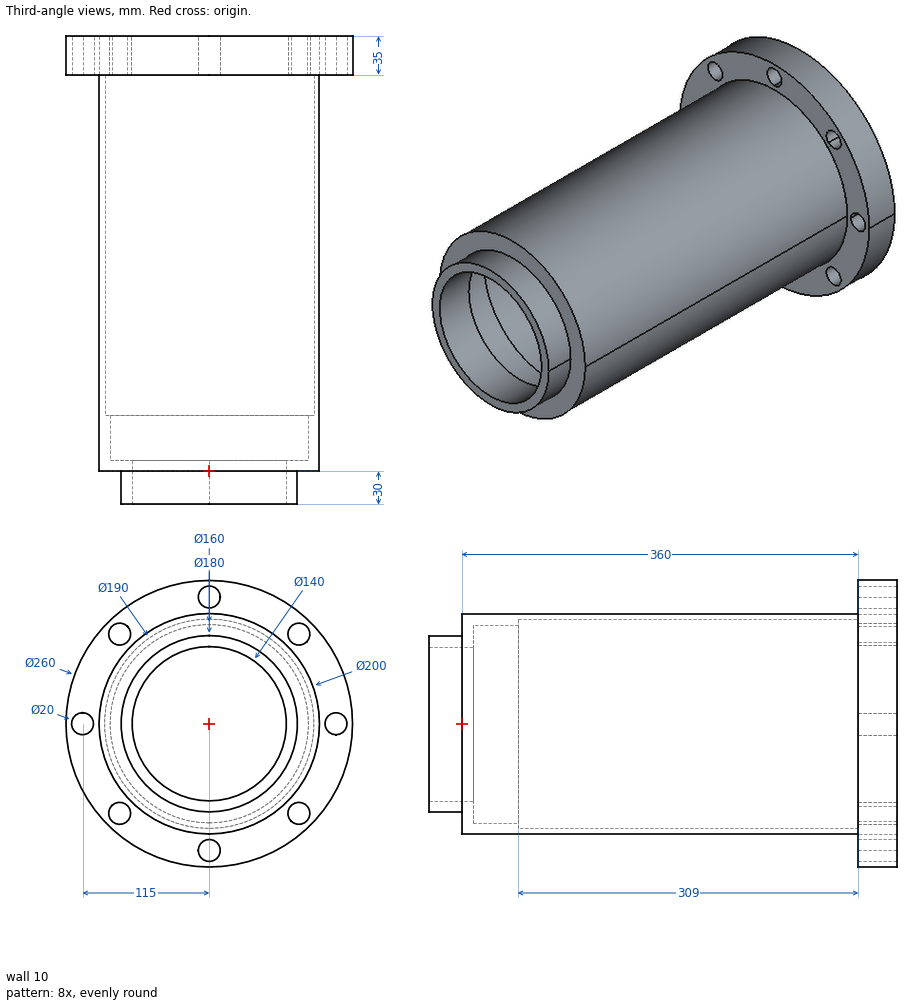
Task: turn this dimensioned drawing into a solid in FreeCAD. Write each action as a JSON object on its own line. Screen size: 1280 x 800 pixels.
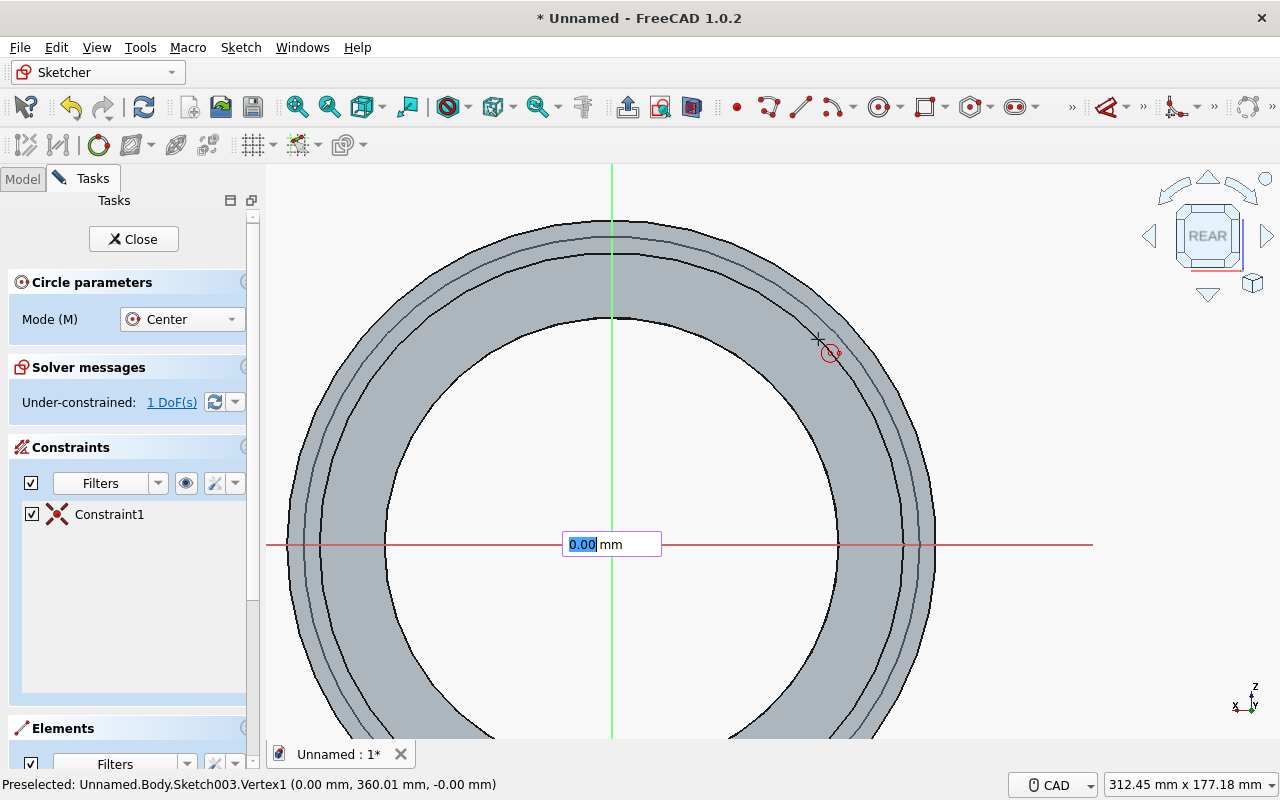
{"action": "left_click", "coordinate": [818, 338]}
{"action": "key", "text": "Escape"}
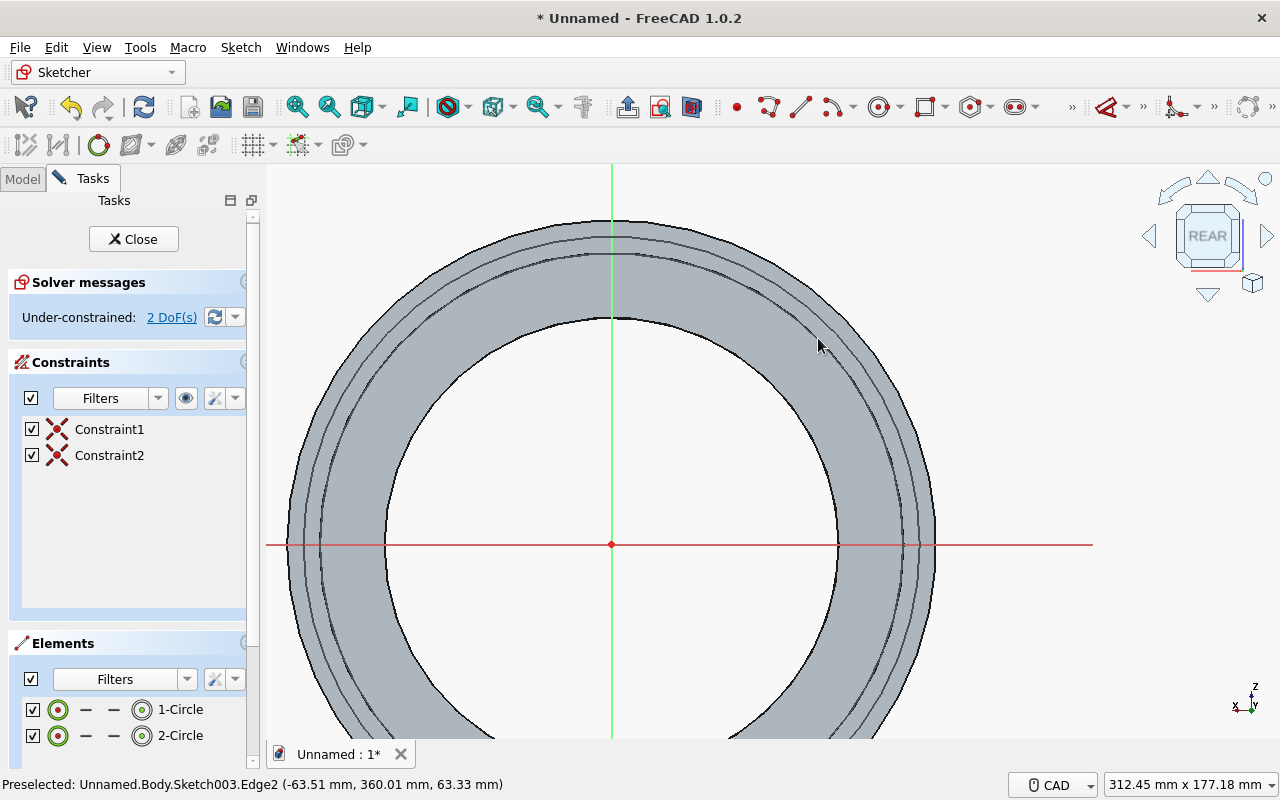
{"action": "left_click", "coordinate": [1106, 108]}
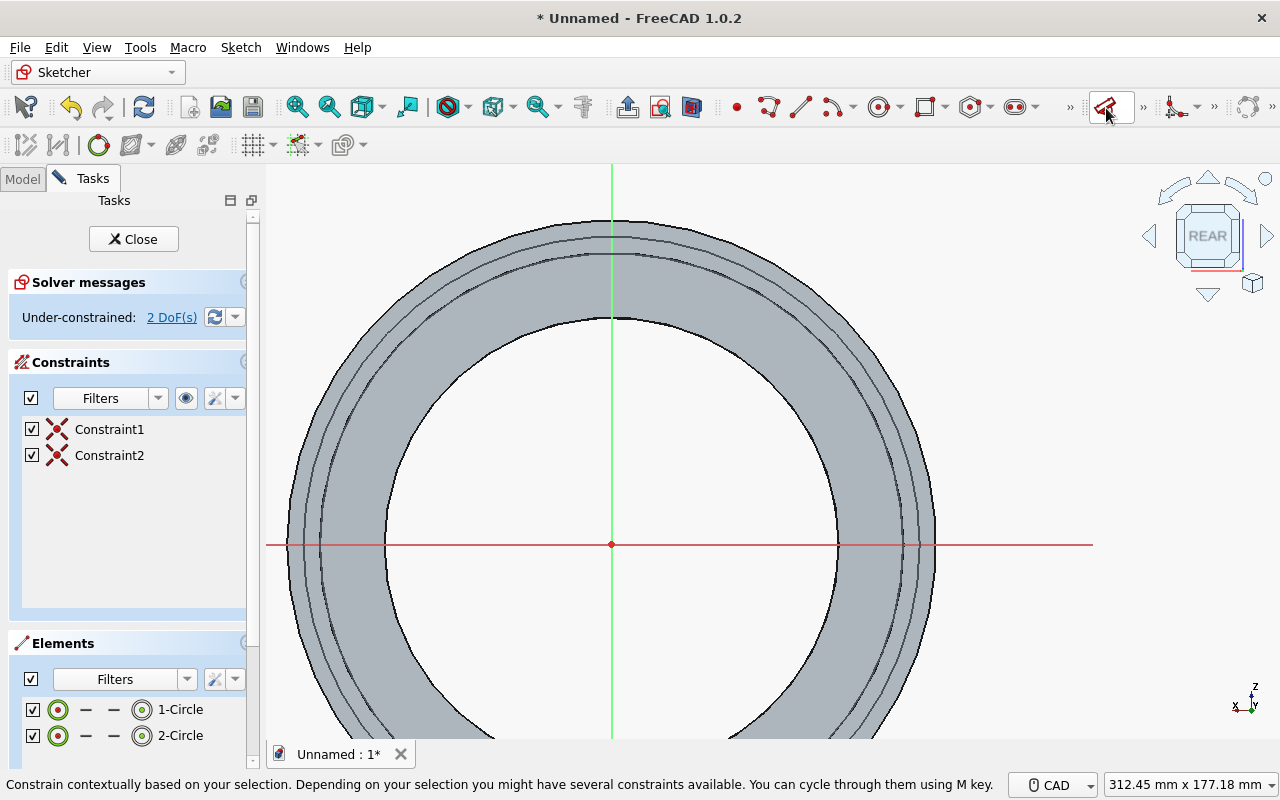
{"action": "left_click", "coordinate": [829, 326]}
{"action": "left_click", "coordinate": [852, 303]}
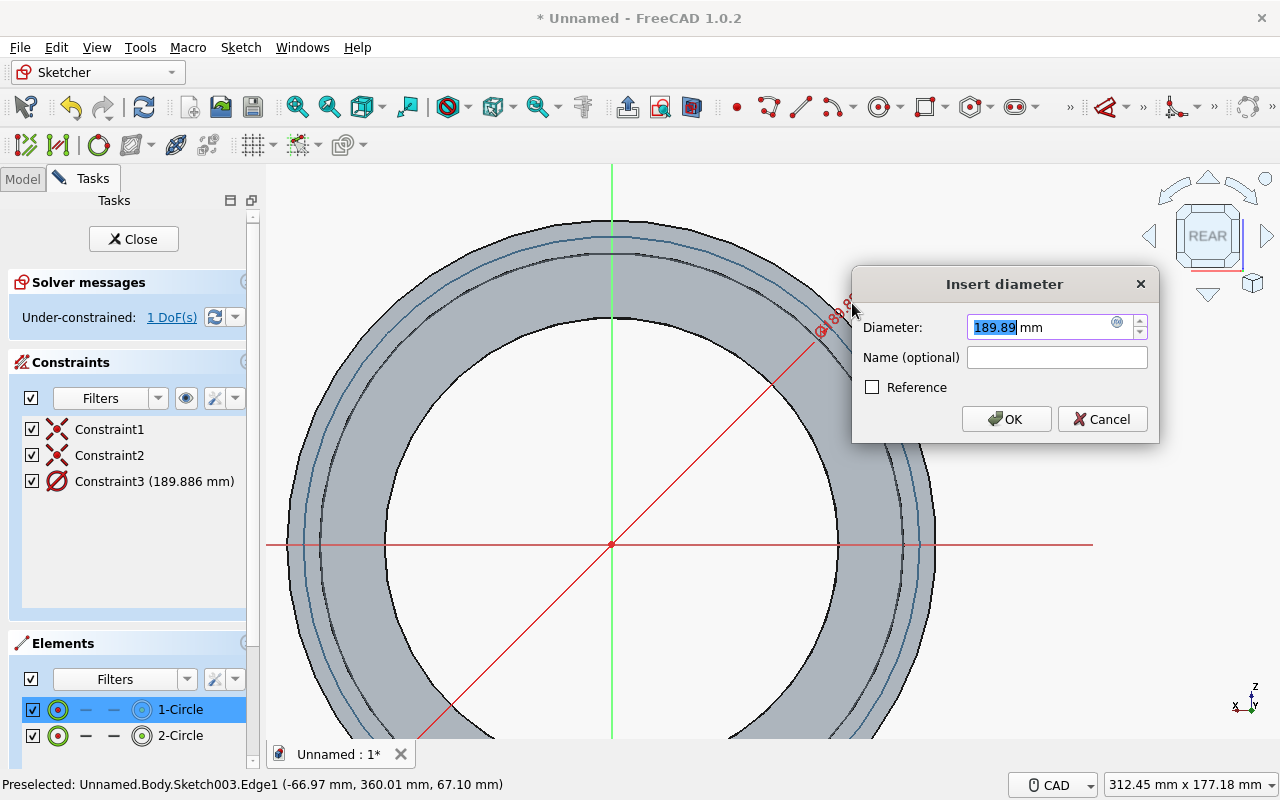
{"action": "type", "text": "190"}
{"action": "key", "text": "Return"}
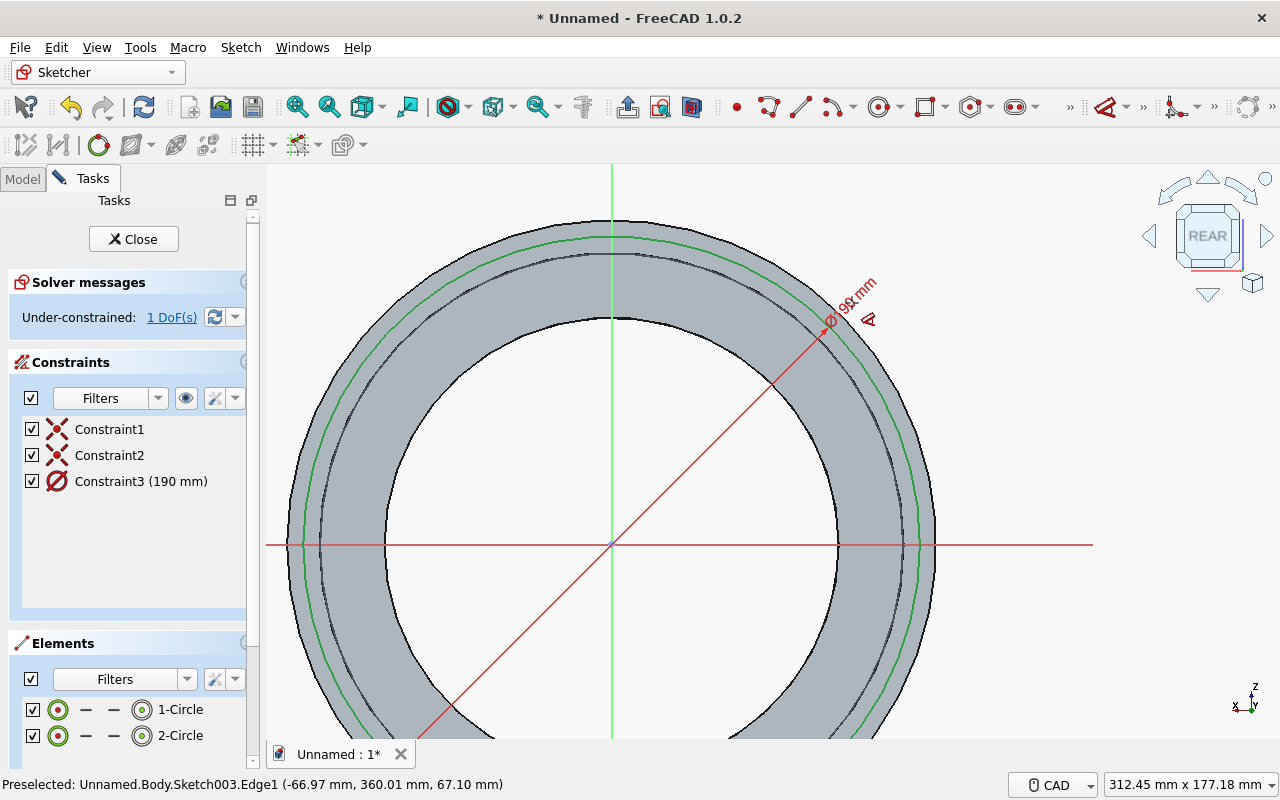
{"action": "left_click", "coordinate": [817, 338]}
{"action": "left_click", "coordinate": [922, 453]}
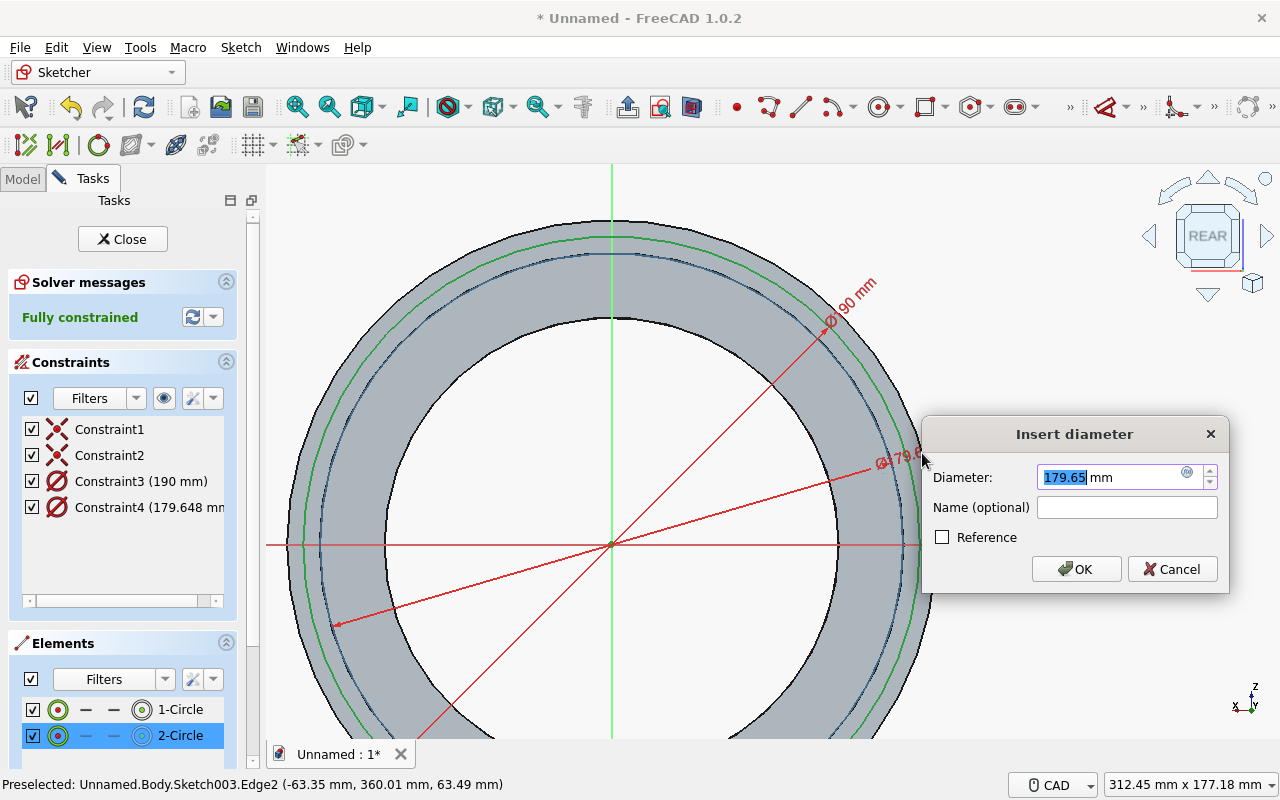
{"action": "type", "text": "180"}
{"action": "key", "text": "Return"}
{"action": "key", "text": "Escape"}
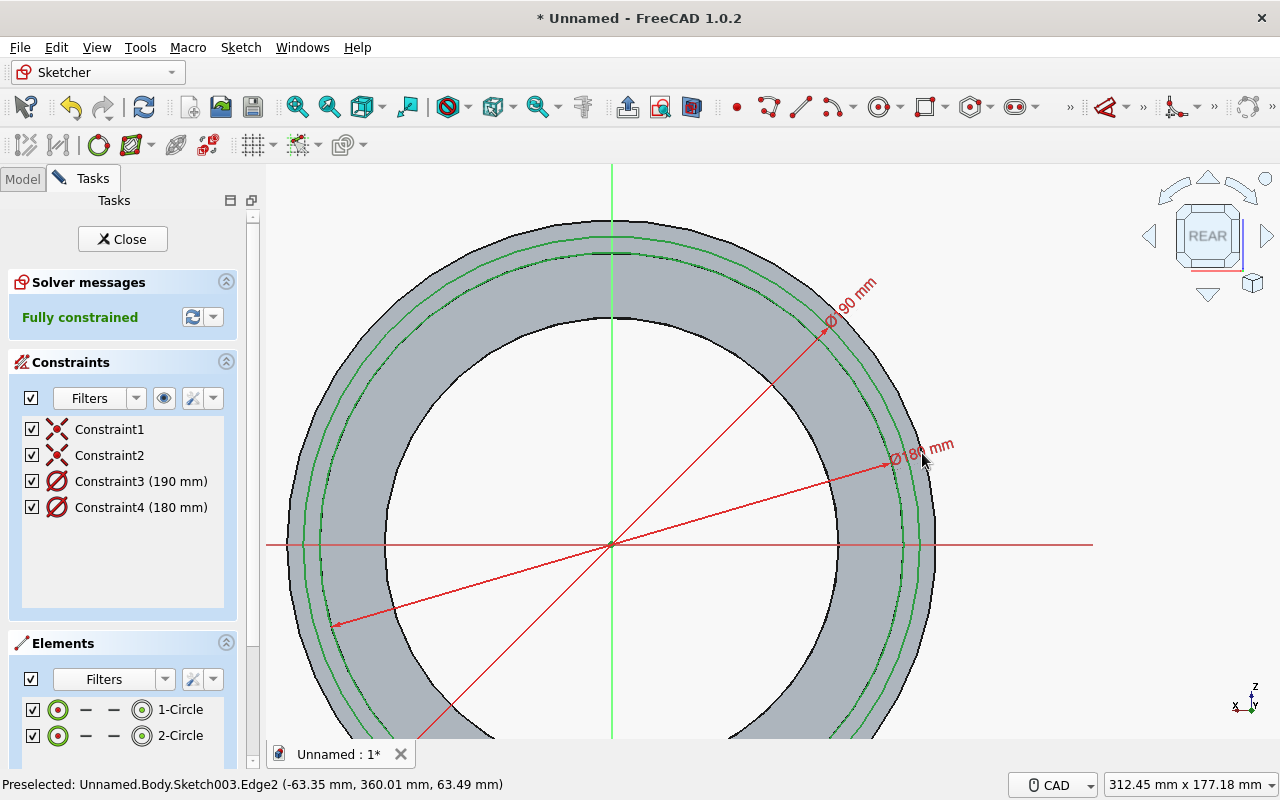
{"action": "left_click", "coordinate": [123, 239]}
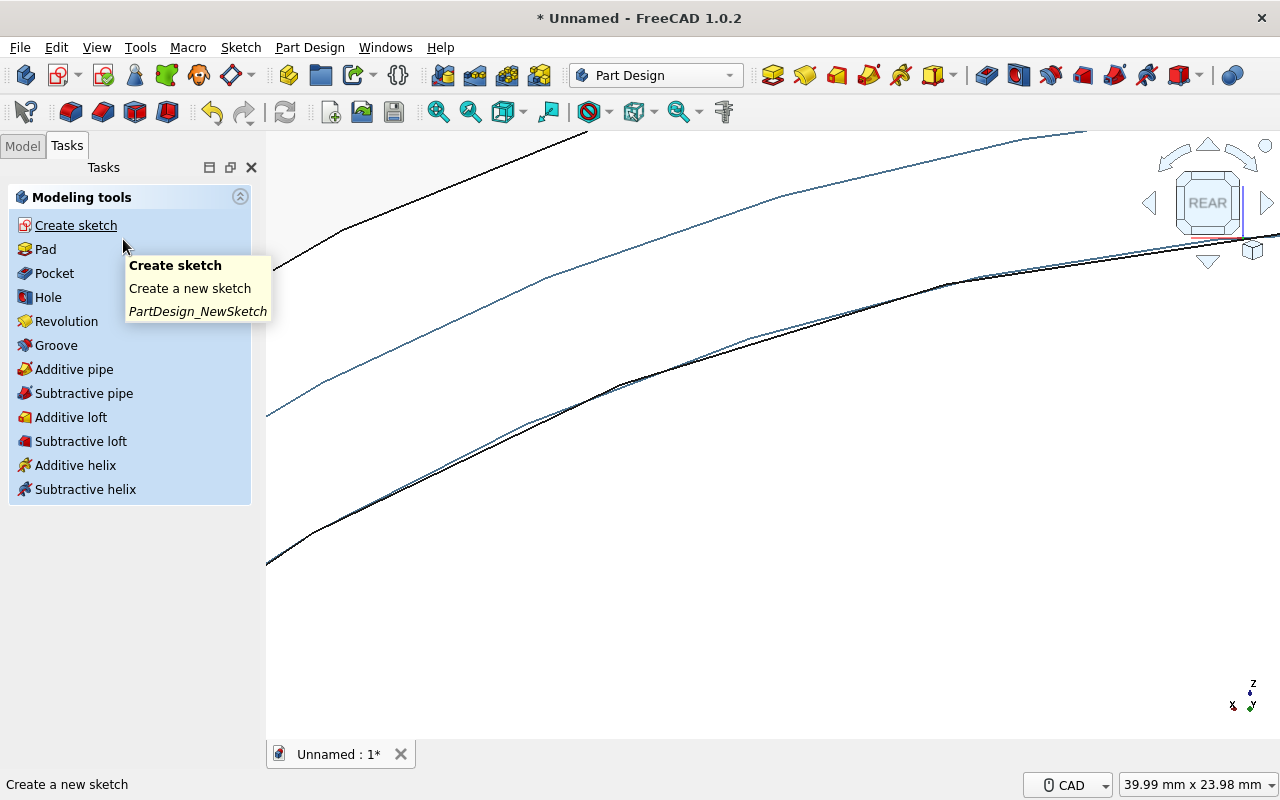
{"action": "left_click", "coordinate": [988, 76]}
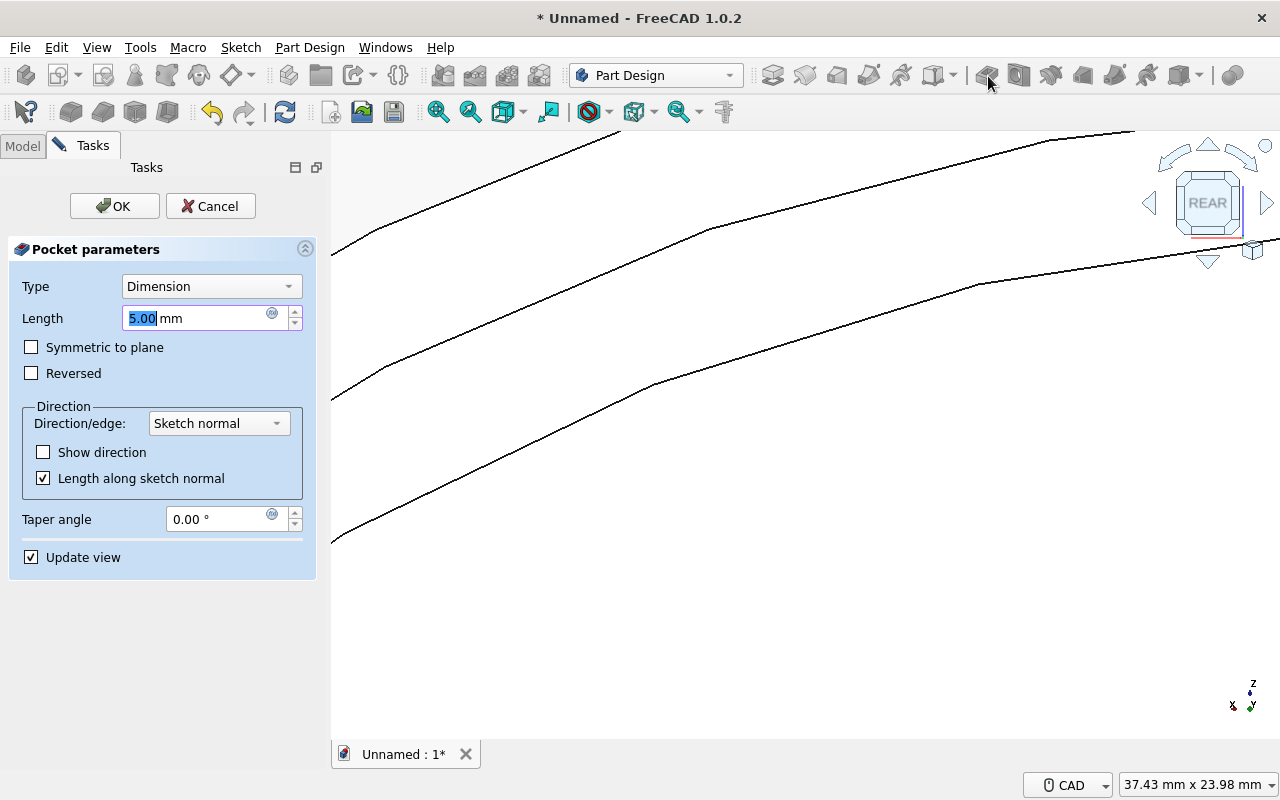
{"action": "left_click", "coordinate": [212, 286]}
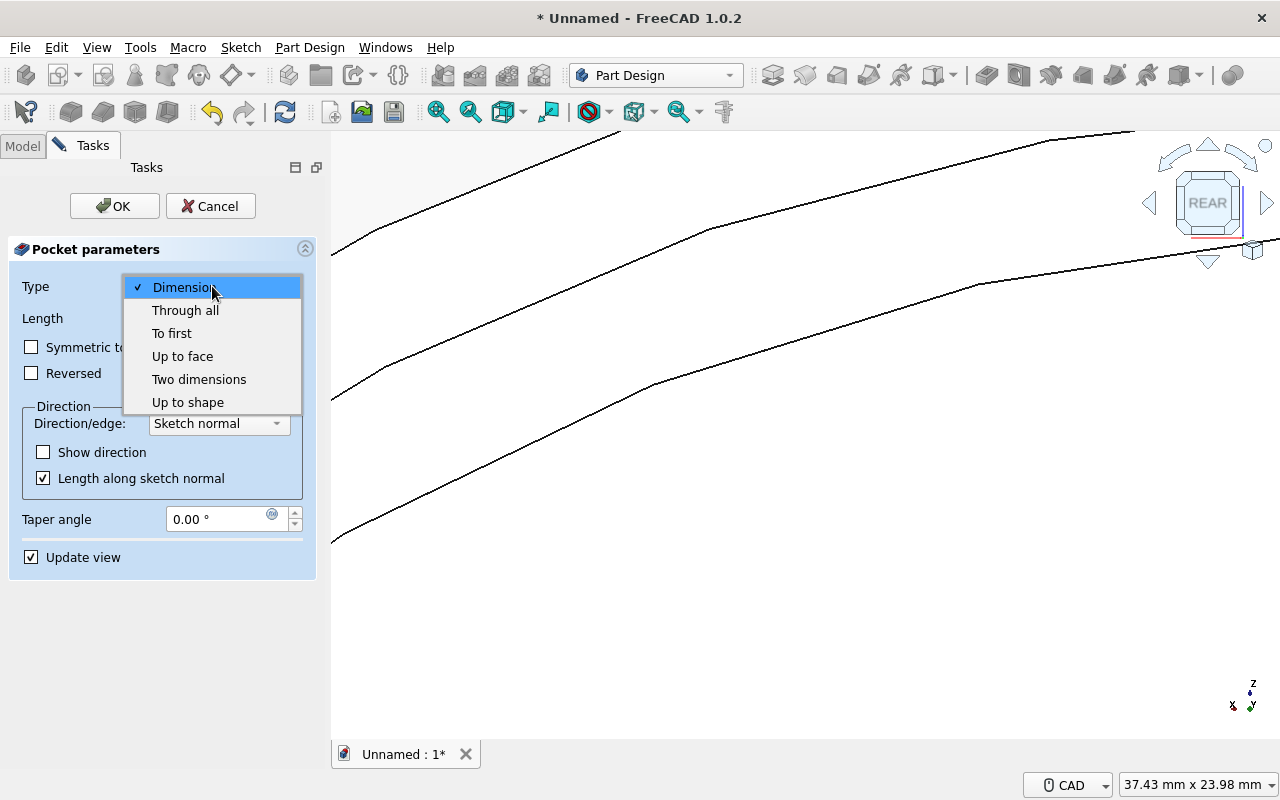
{"action": "left_click", "coordinate": [212, 380]}